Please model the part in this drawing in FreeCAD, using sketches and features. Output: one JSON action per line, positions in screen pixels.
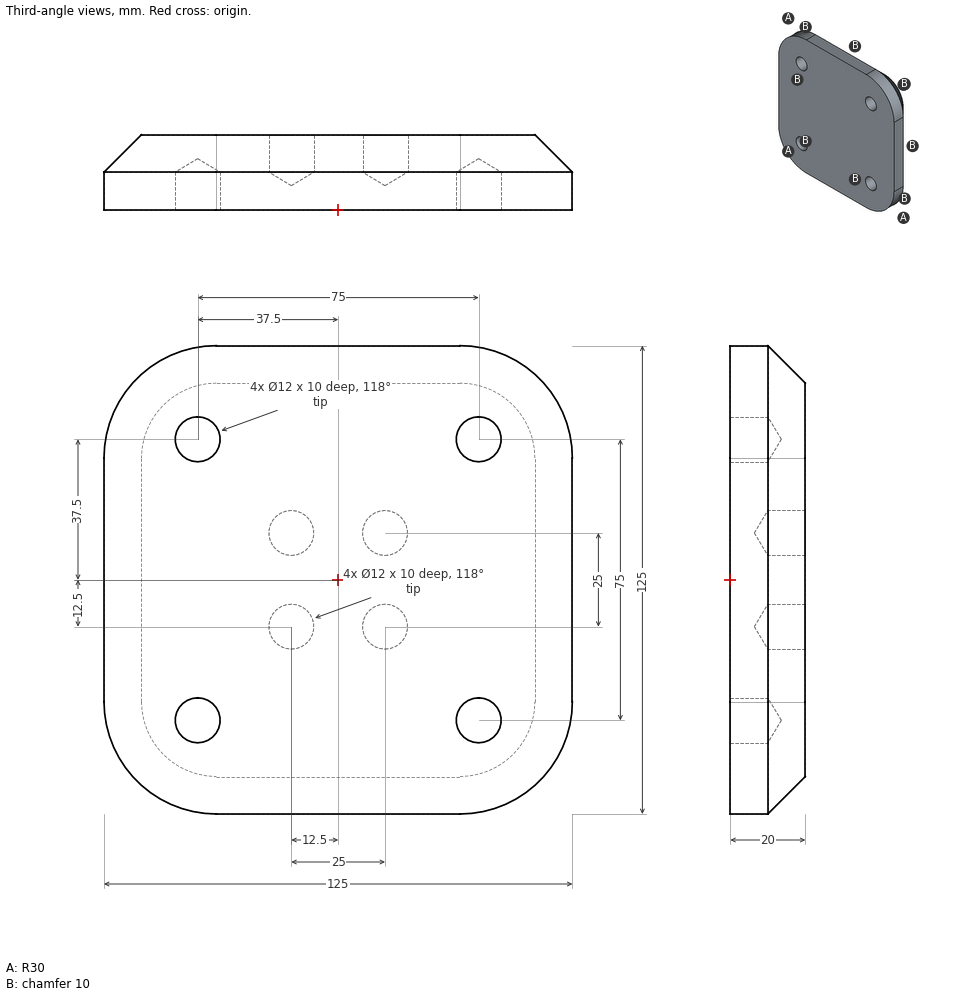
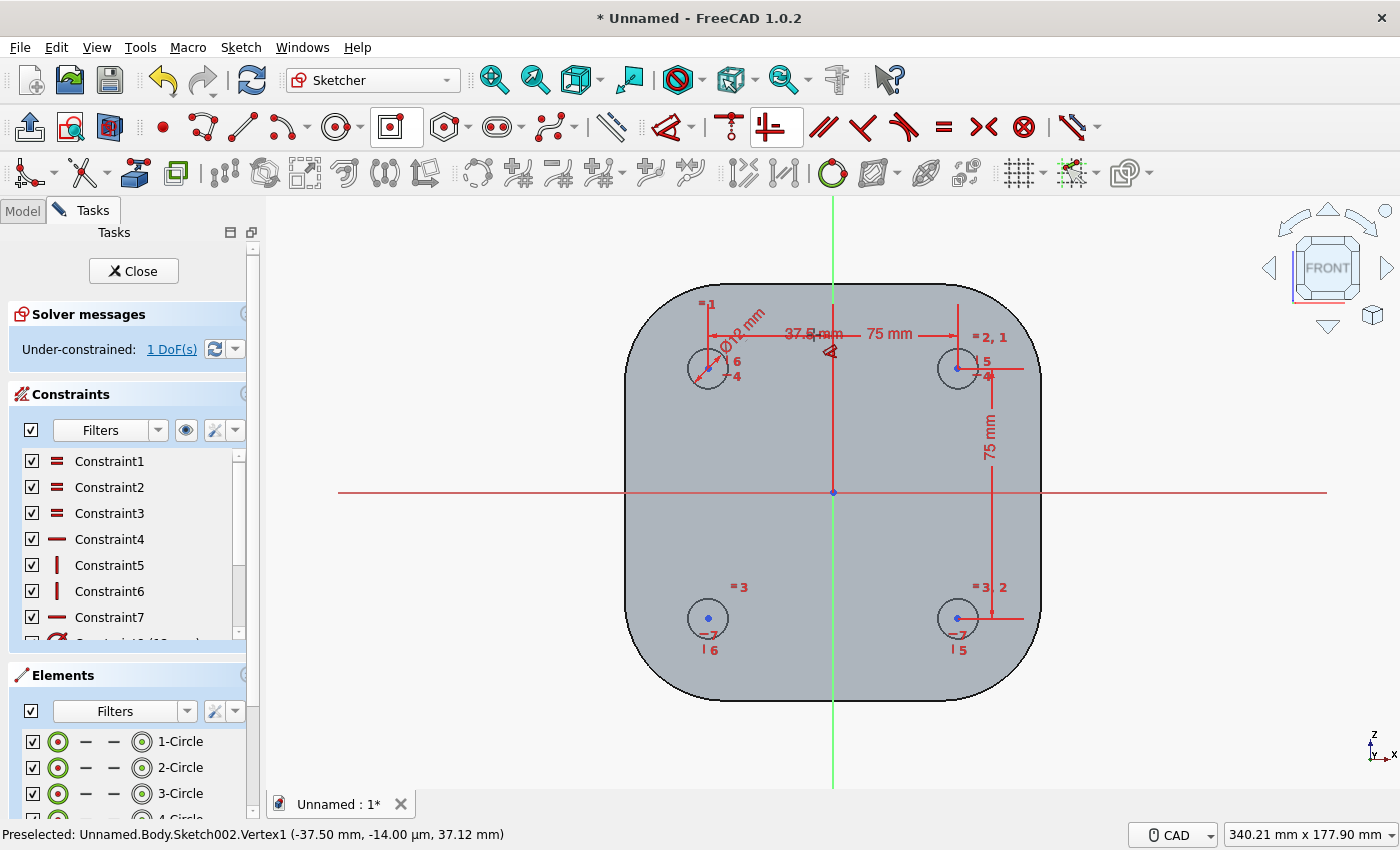
{"action": "left_click", "coordinate": [708, 369]}
{"action": "left_click", "coordinate": [674, 431]}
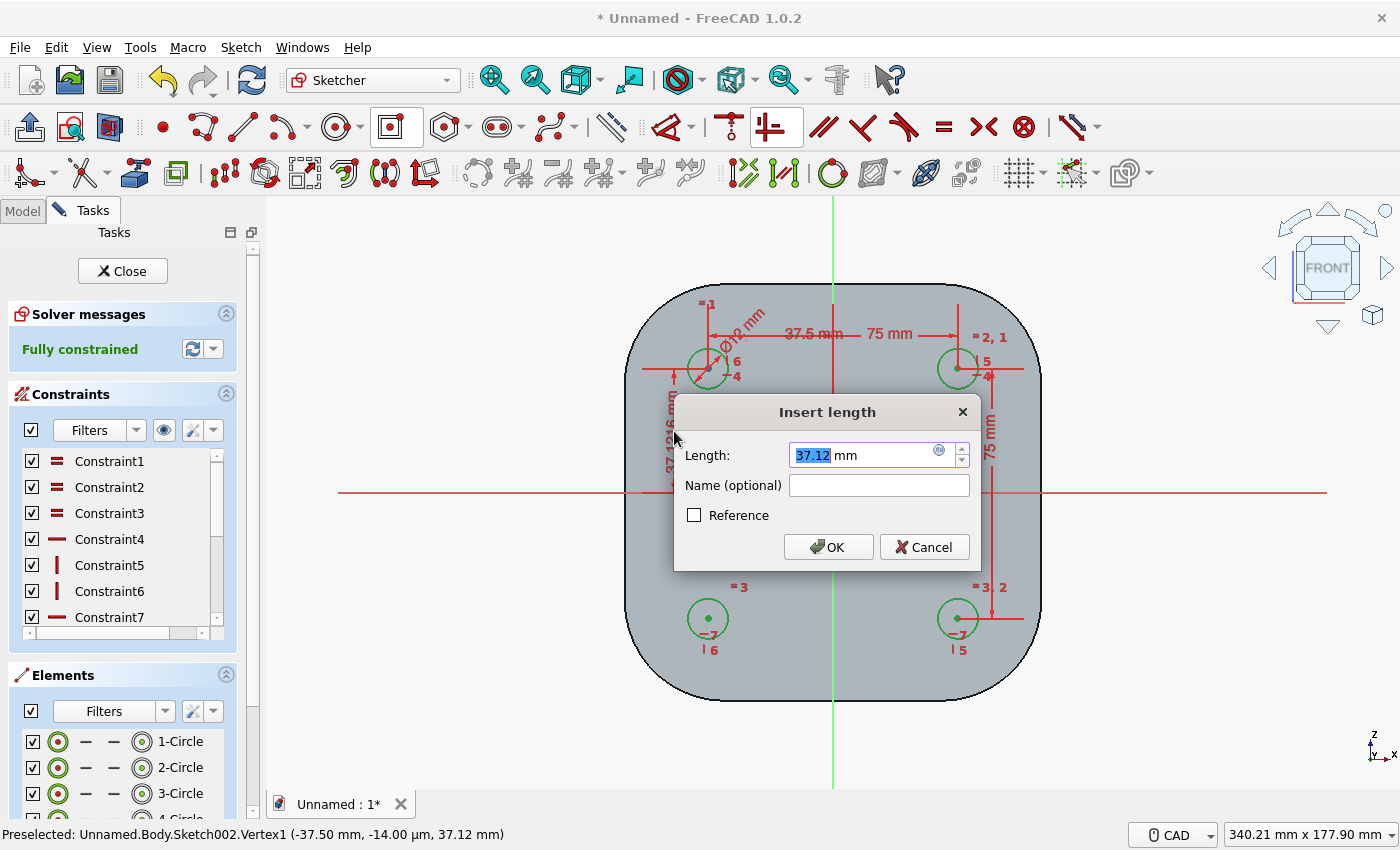
{"action": "type", "text": "37.5"}
{"action": "key", "text": "Return"}
{"action": "key", "text": "Escape"}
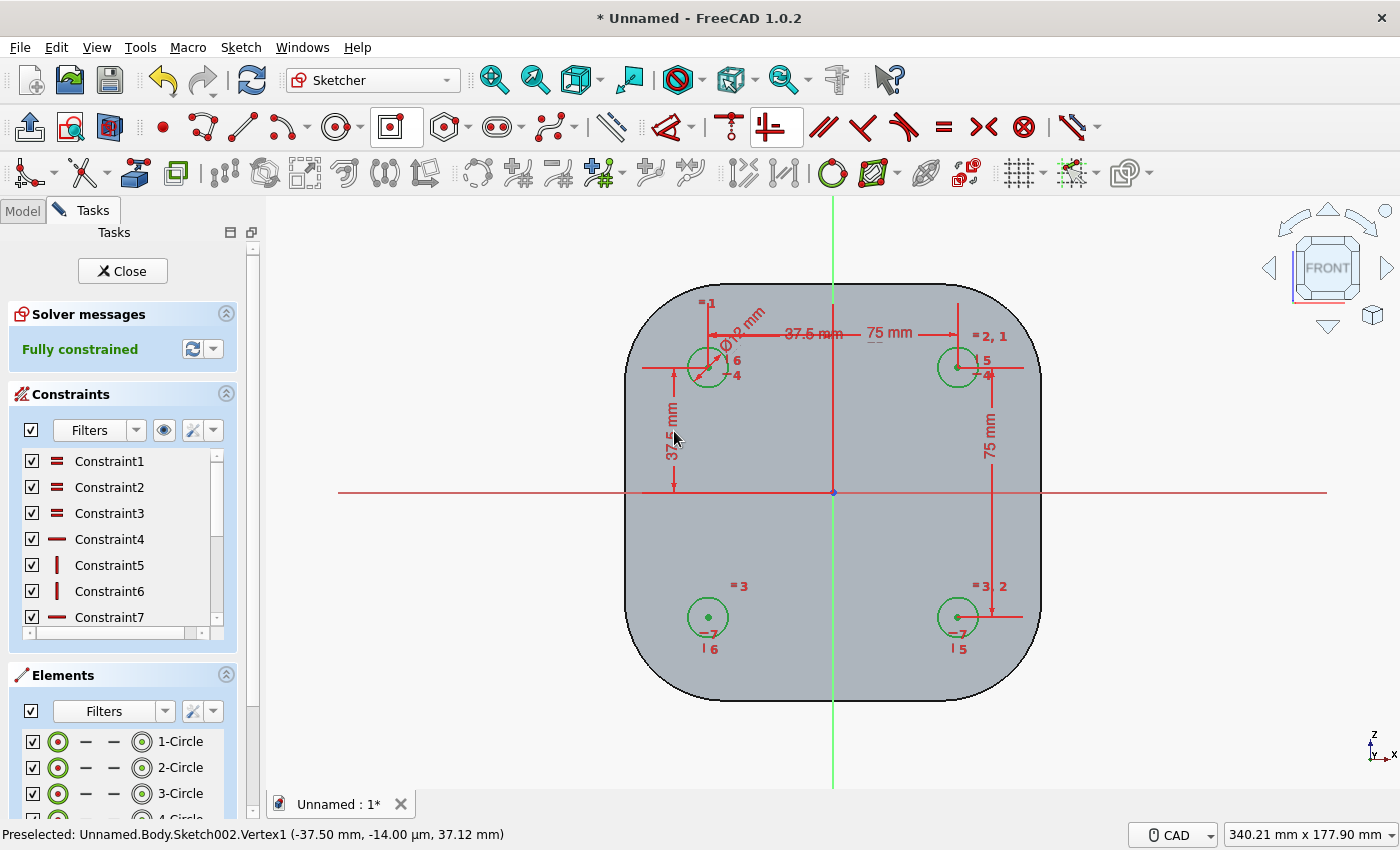
{"action": "left_click", "coordinate": [123, 271]}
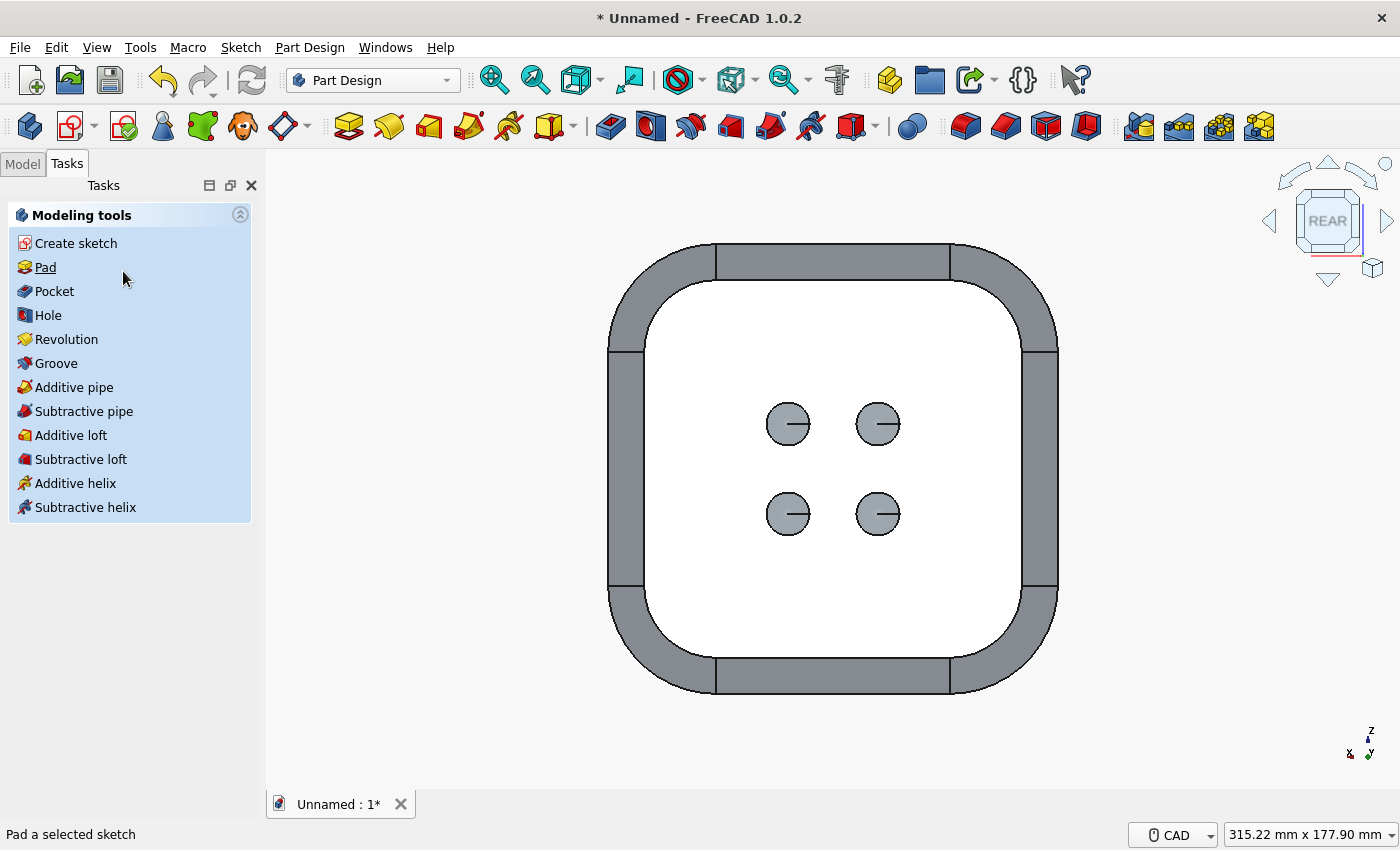
{"action": "left_click", "coordinate": [652, 126]}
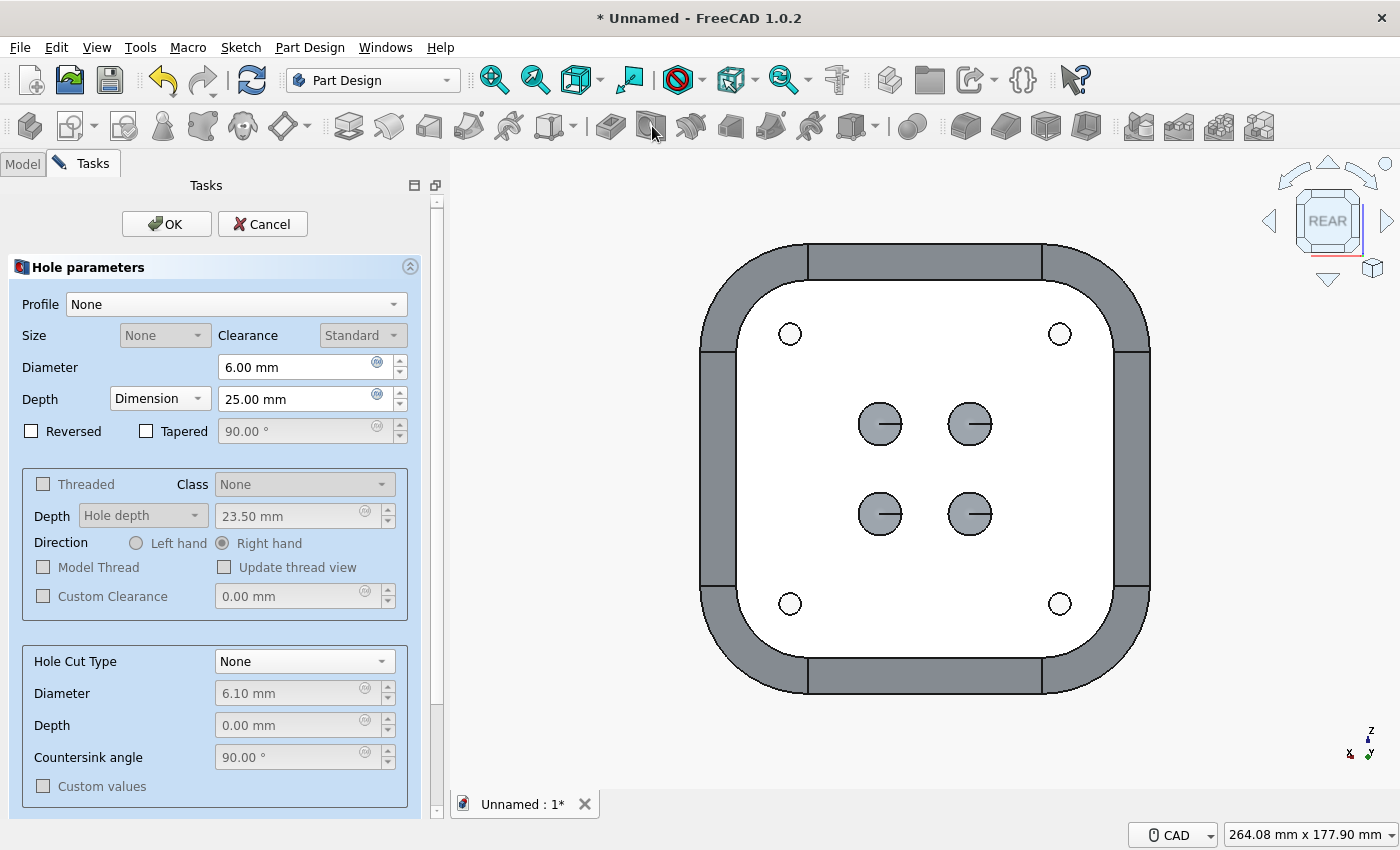
{"action": "triple_click", "coordinate": [305, 367]}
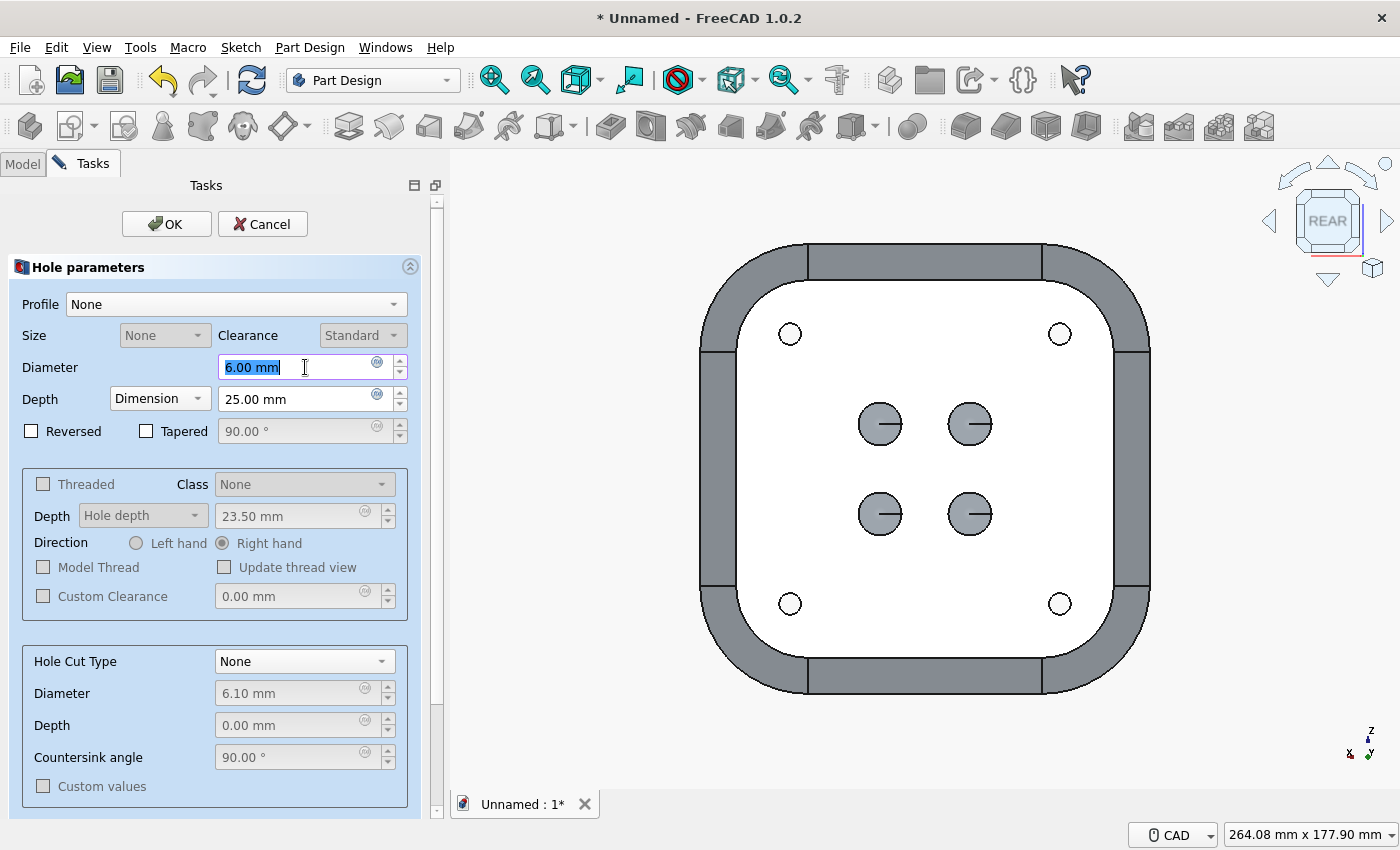
{"action": "type", "text": "12"}
{"action": "key", "text": "Tab"}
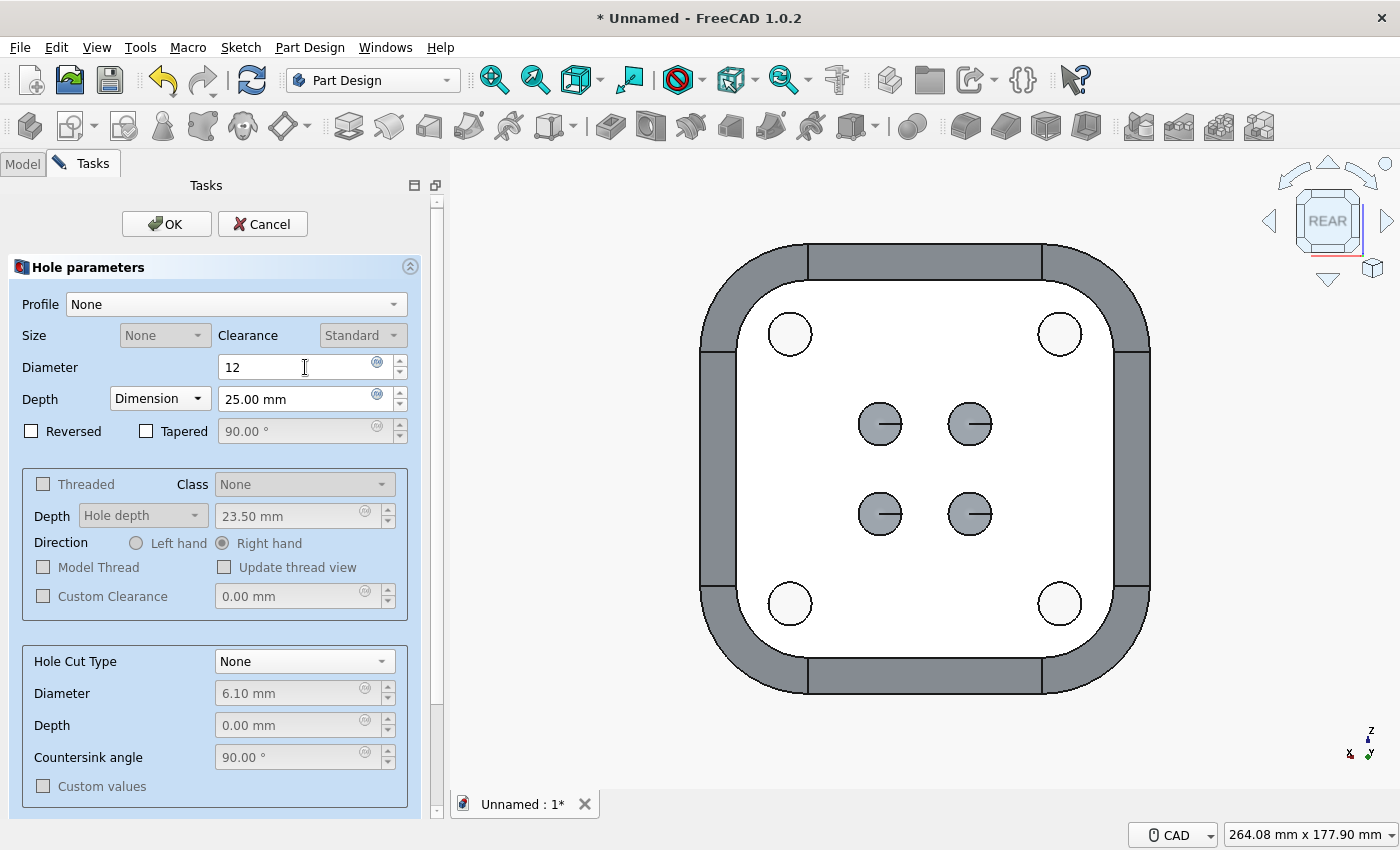
{"action": "triple_click", "coordinate": [305, 399]}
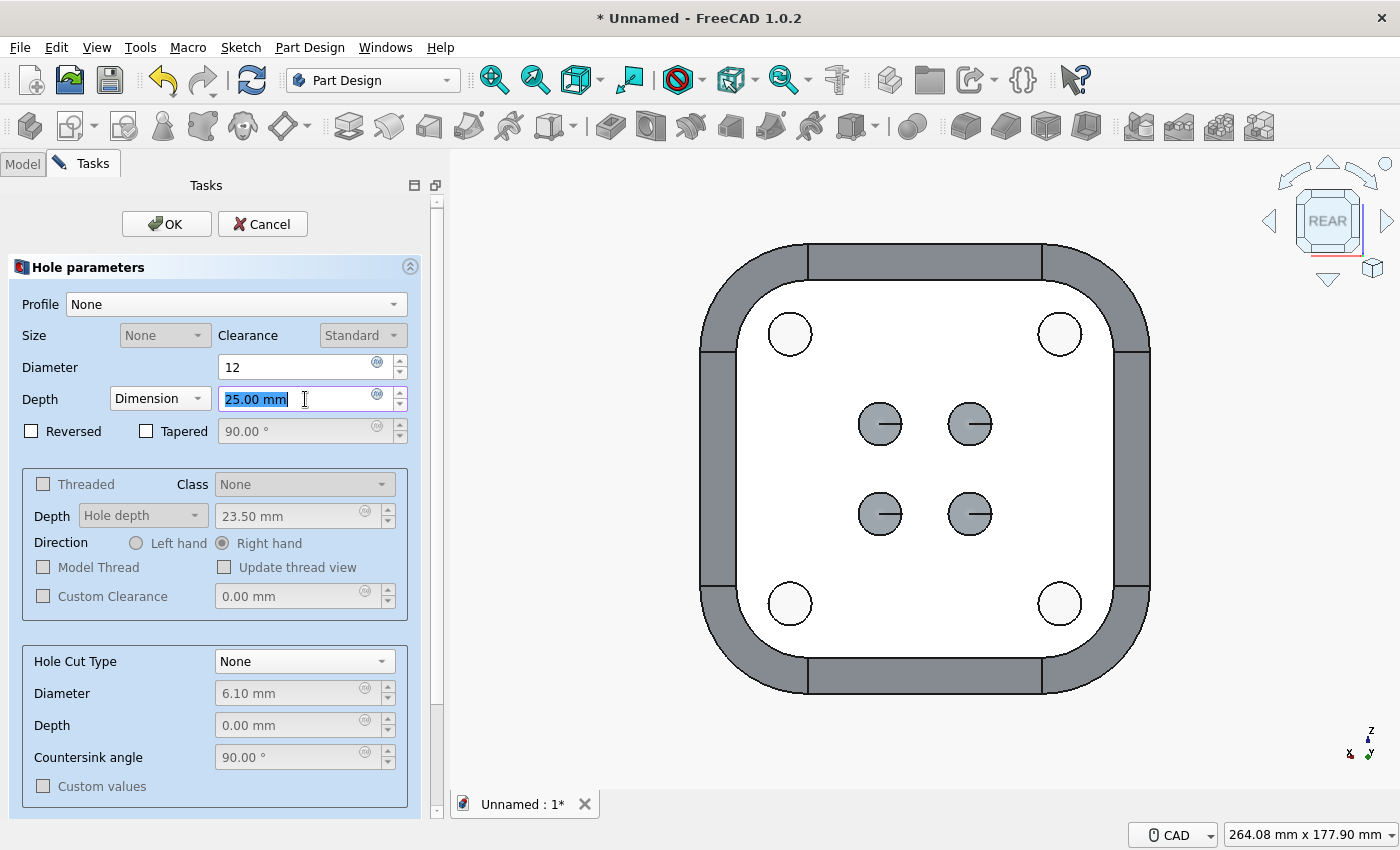
{"action": "type", "text": "10"}
{"action": "key", "text": "Tab"}